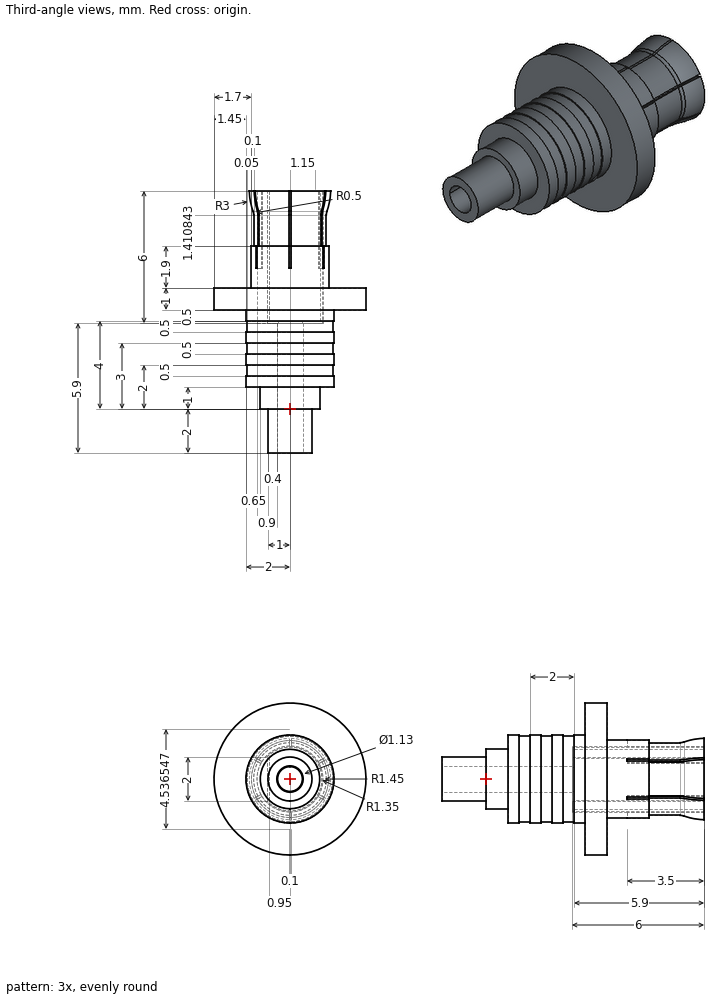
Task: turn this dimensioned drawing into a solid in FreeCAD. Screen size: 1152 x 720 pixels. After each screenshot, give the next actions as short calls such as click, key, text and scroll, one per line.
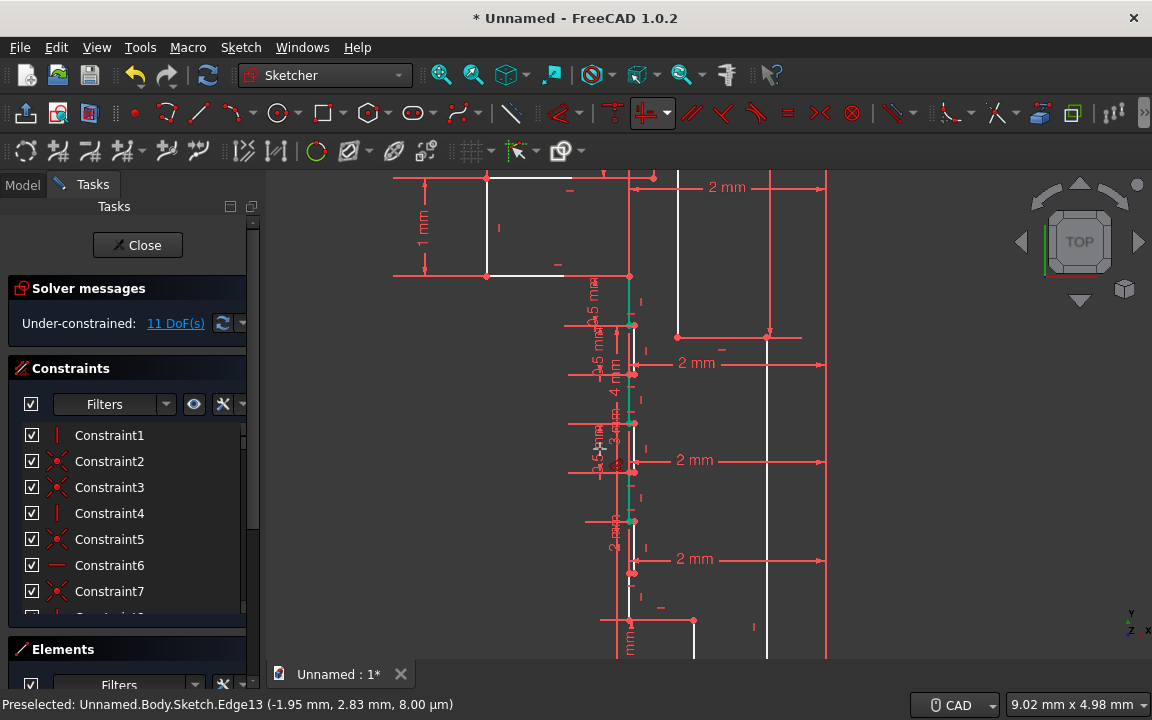
click(634, 537)
click(600, 559)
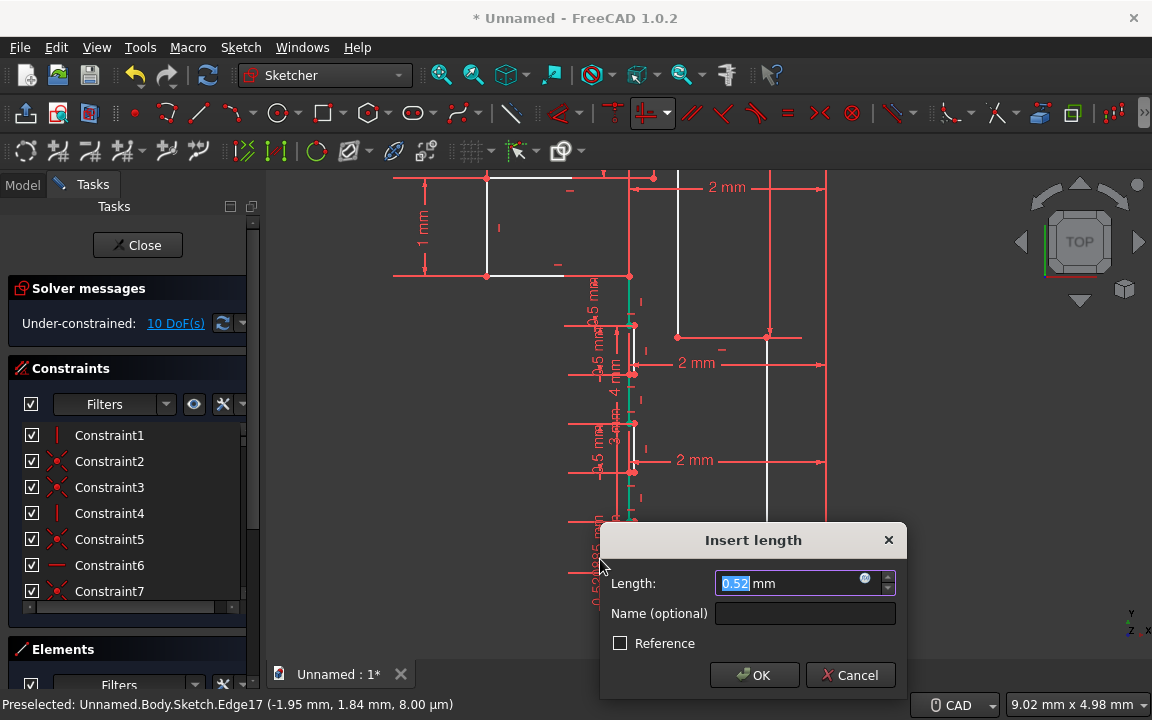
text(0.5)
key(Return)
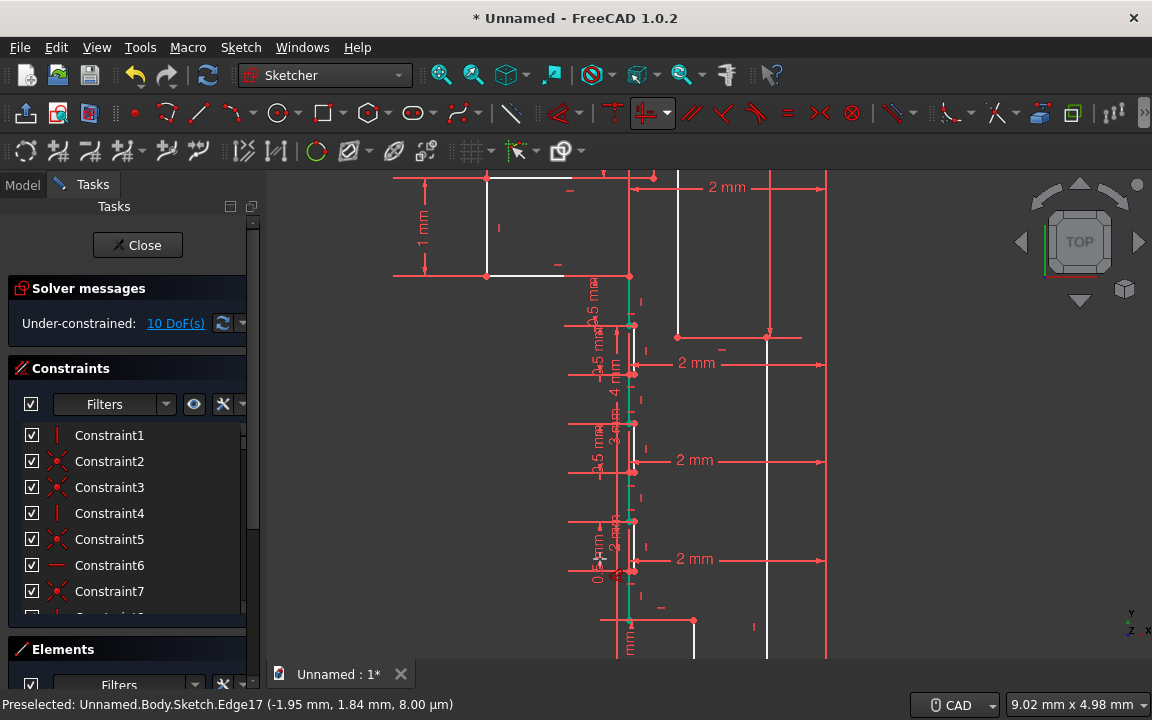
scroll(635, 442, down, 7)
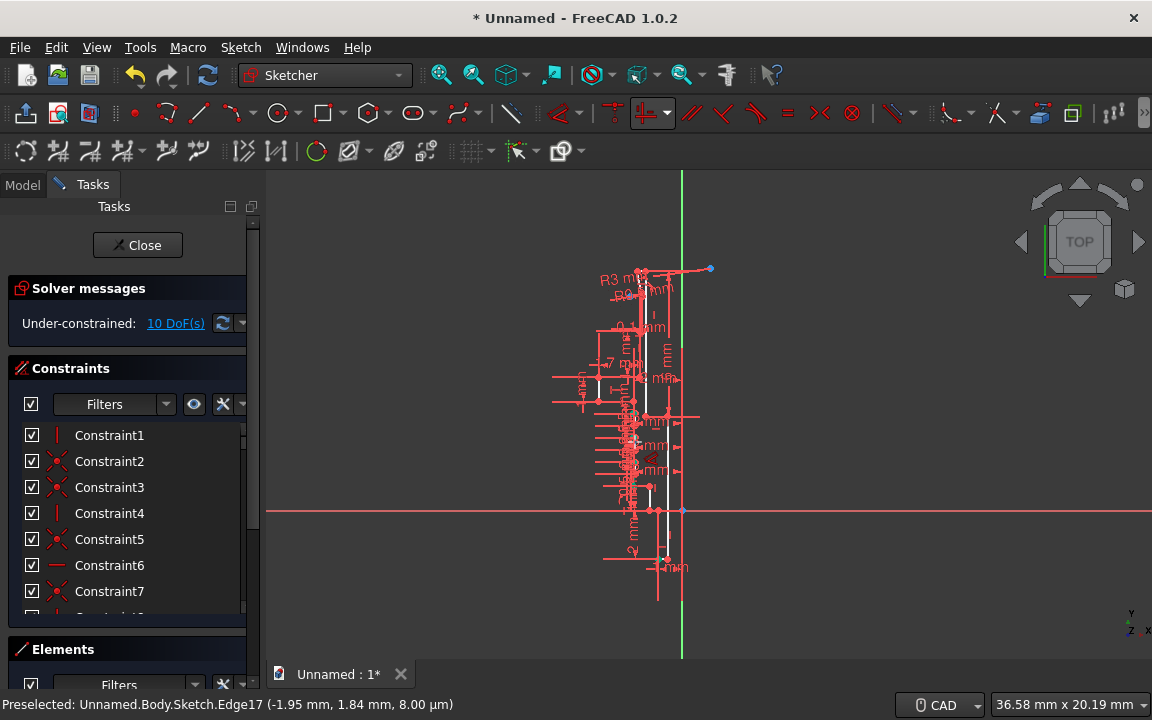
scroll(661, 559, up, 8)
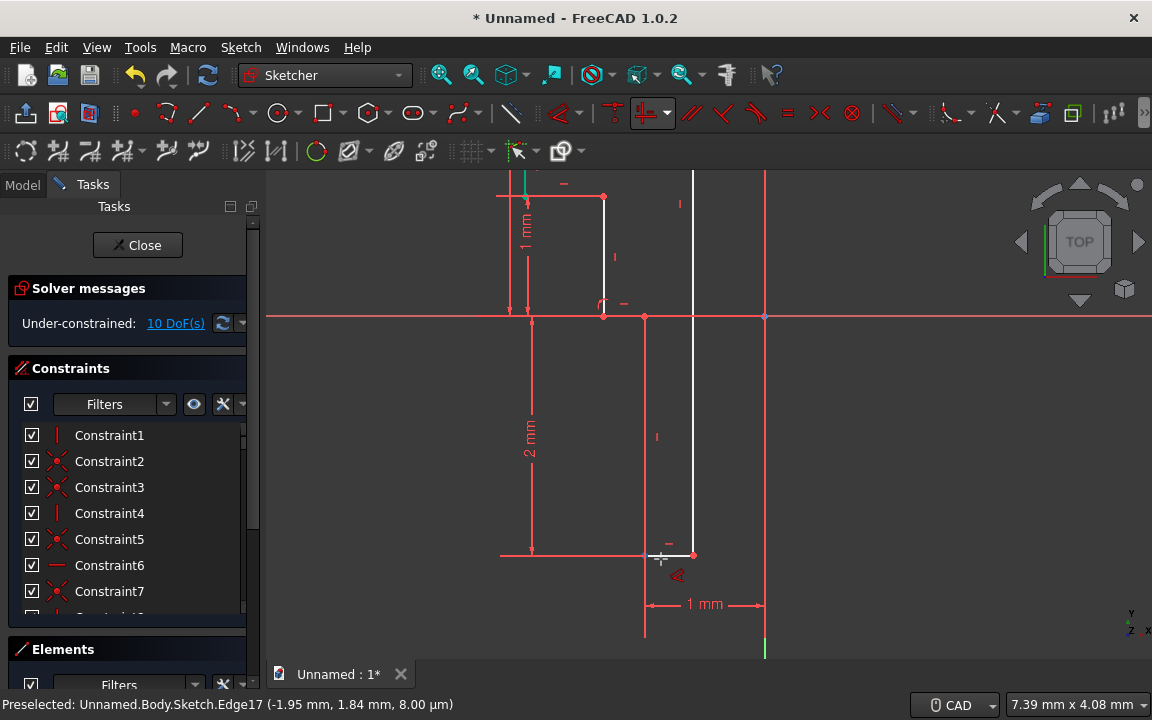
click(659, 556)
click(669, 522)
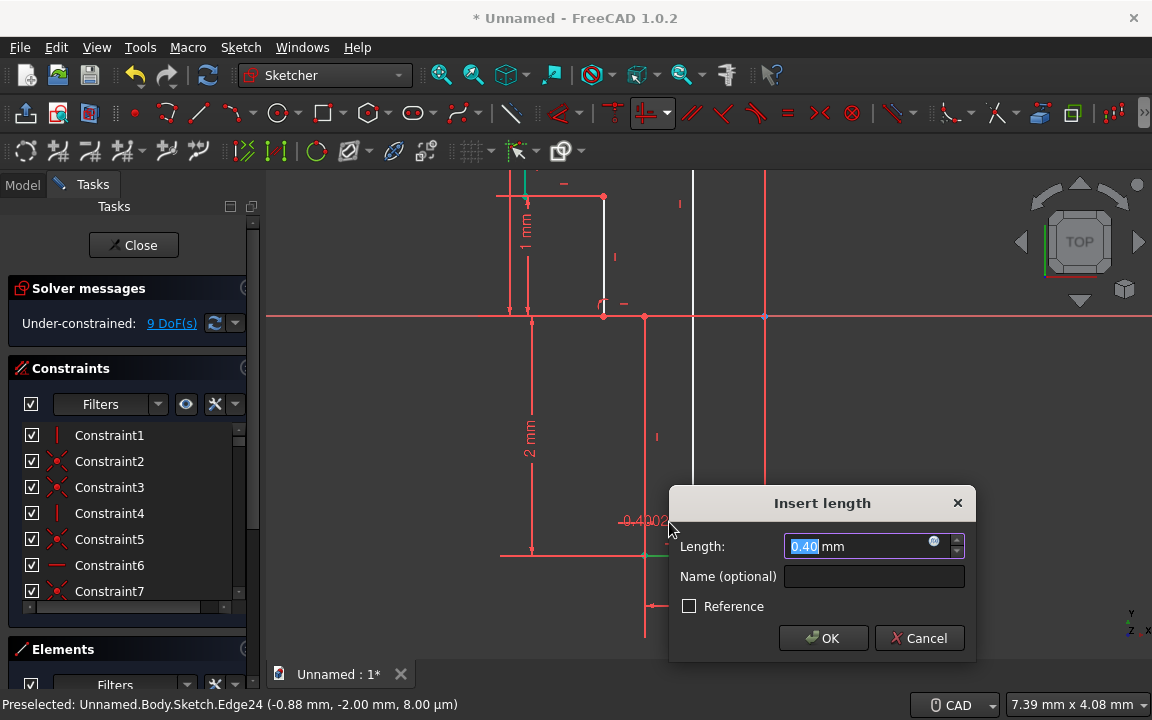
text(0.4)
key(Return)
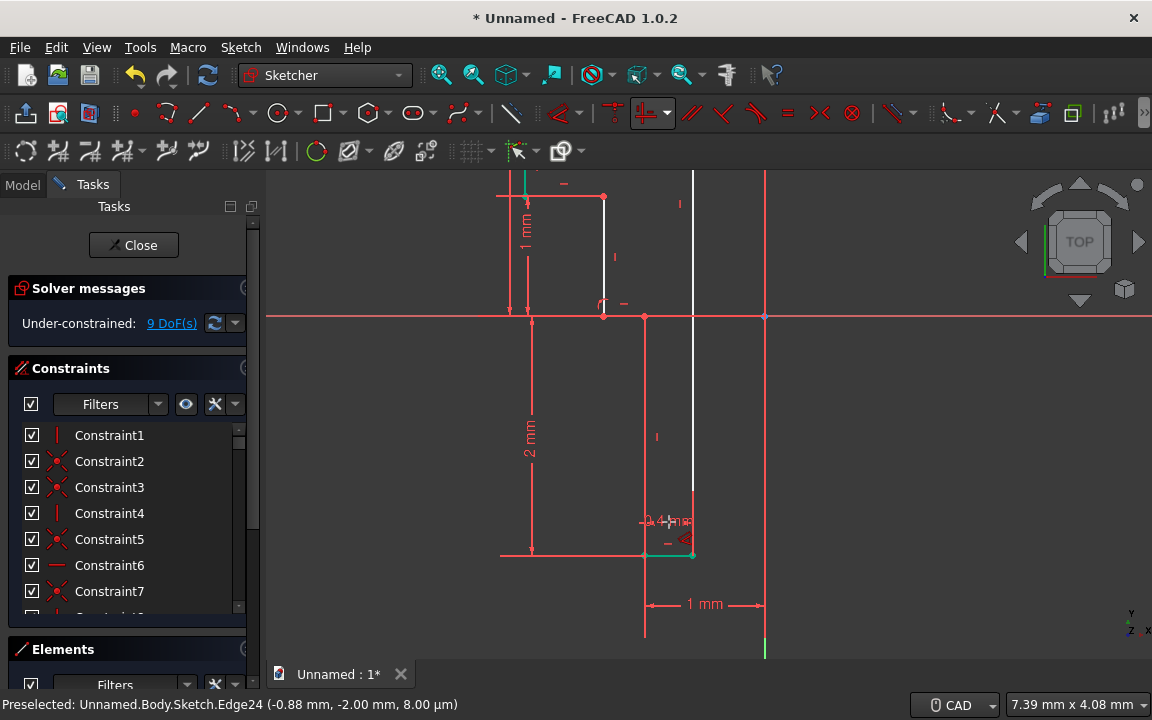
click(693, 344)
click(727, 377)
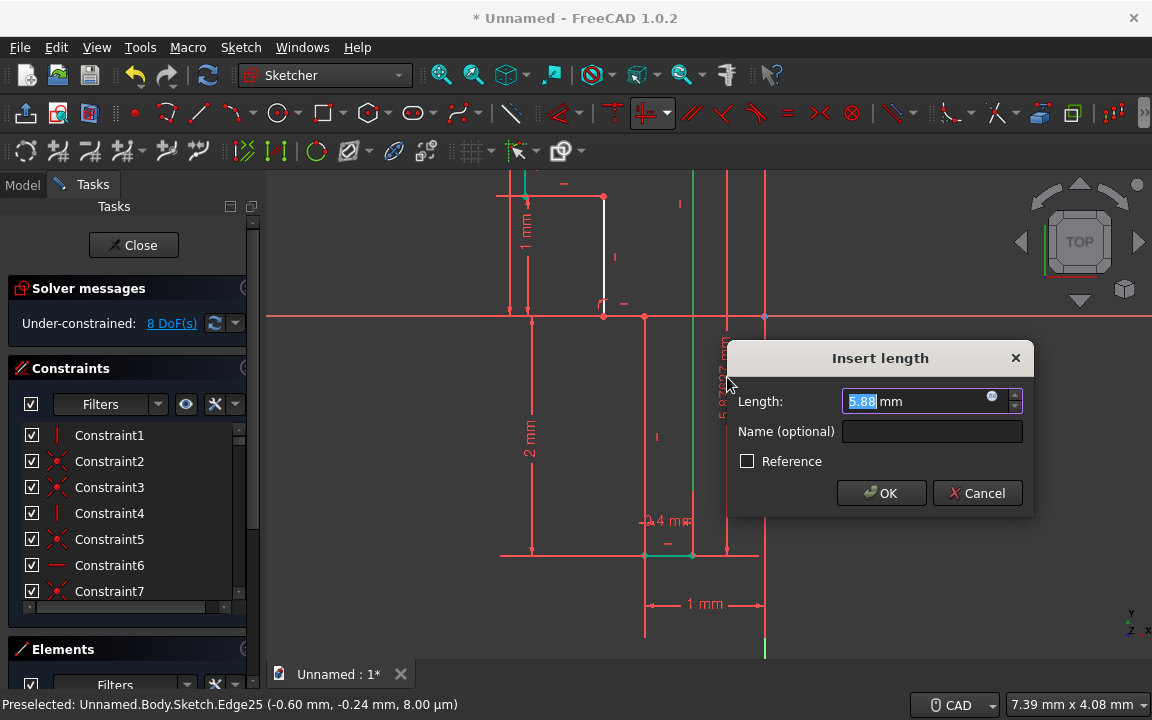
text(5.9)
key(Return)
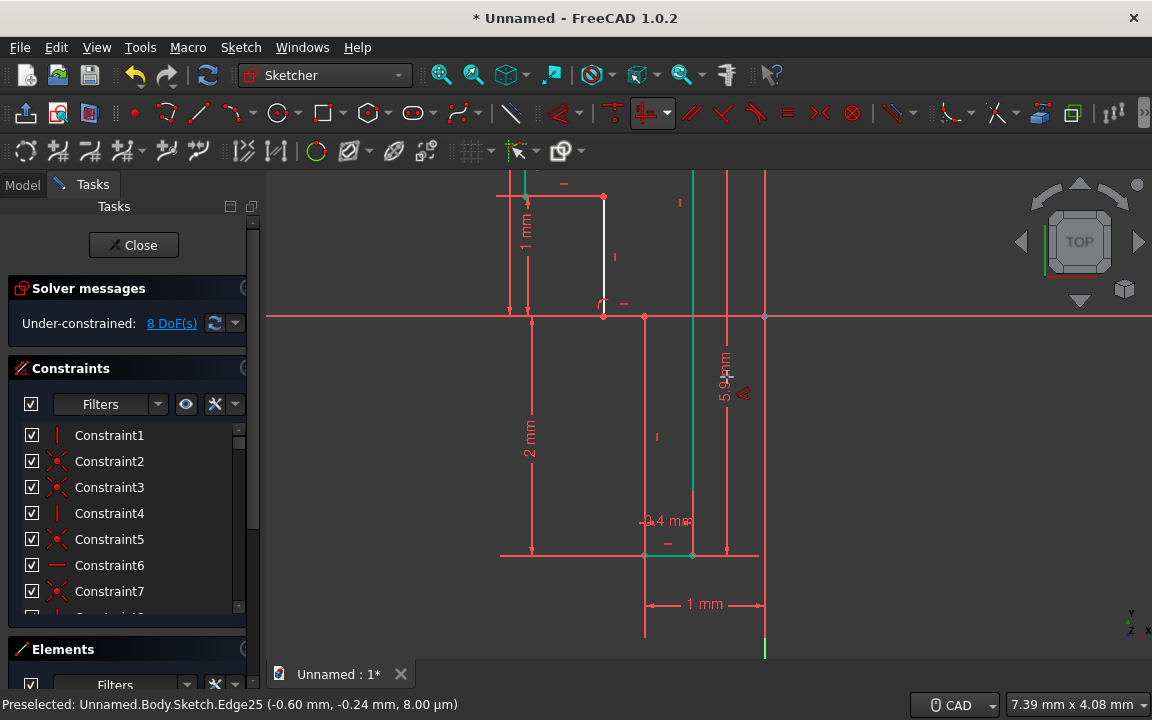
scroll(661, 559, down, 8)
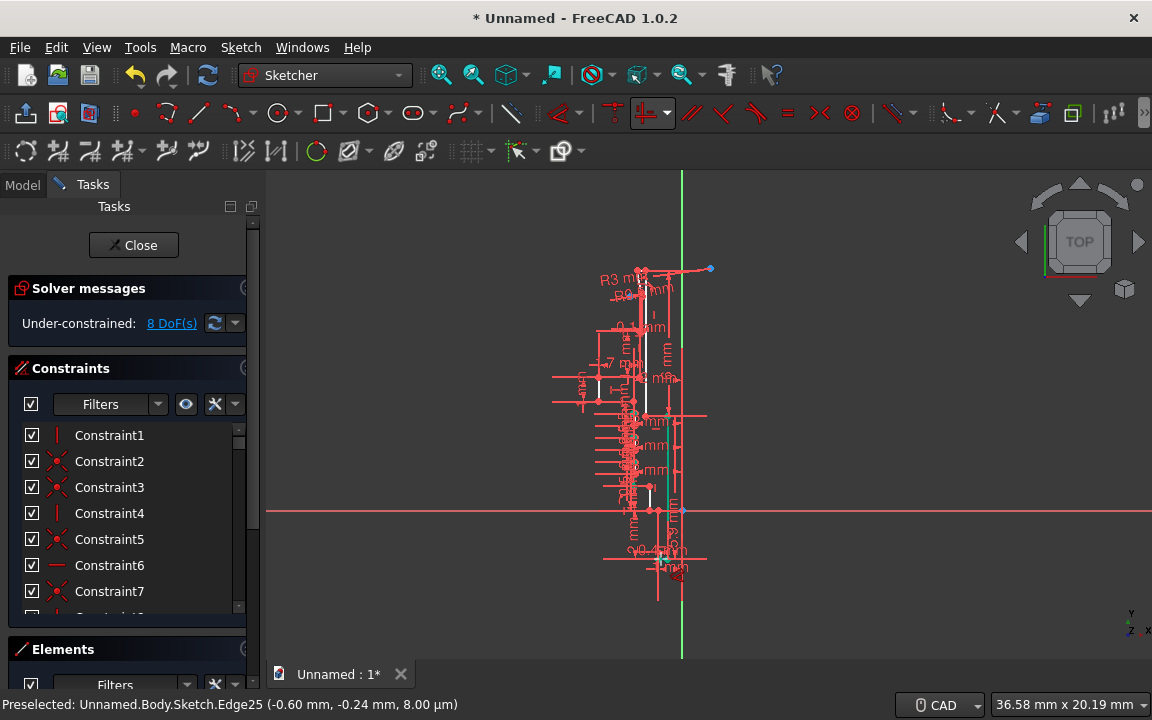
scroll(661, 416, up, 4)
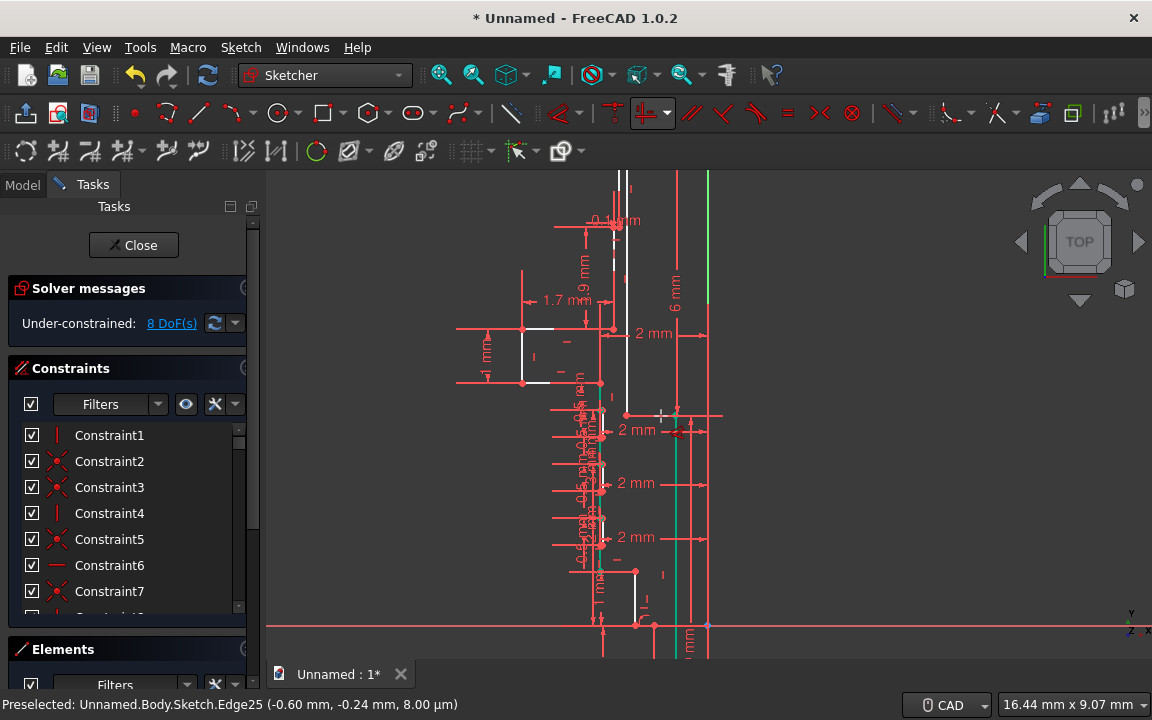
click(661, 416)
click(662, 382)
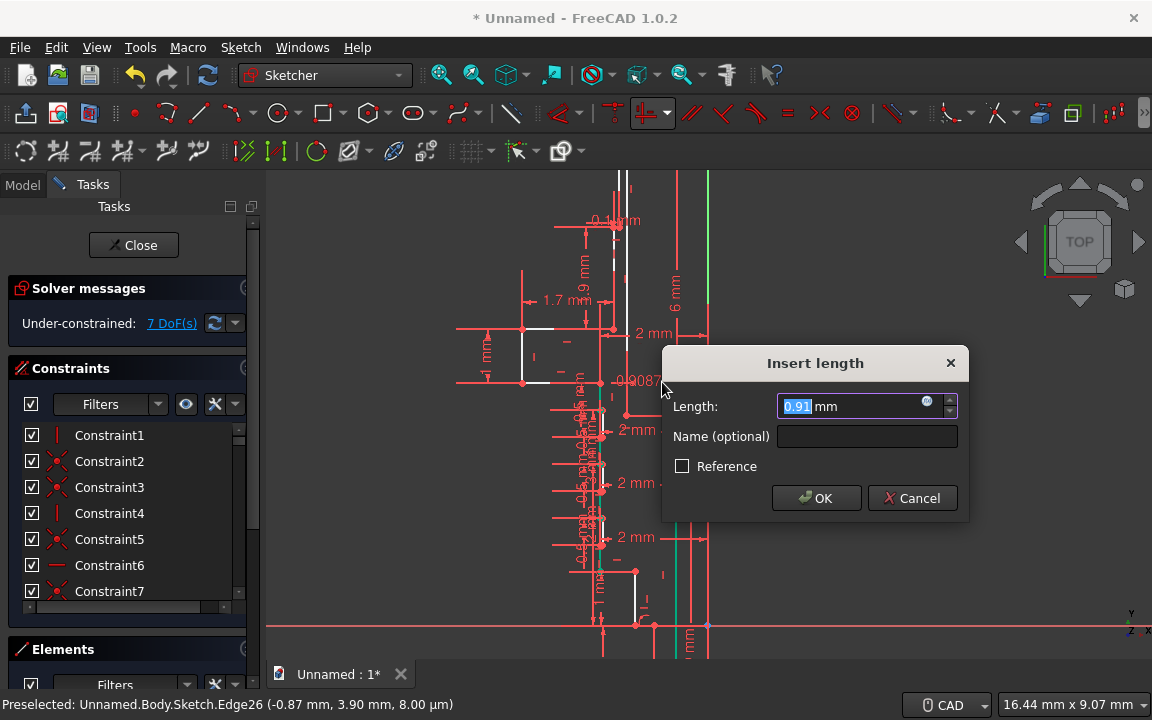
text(0.9)
key(Return)